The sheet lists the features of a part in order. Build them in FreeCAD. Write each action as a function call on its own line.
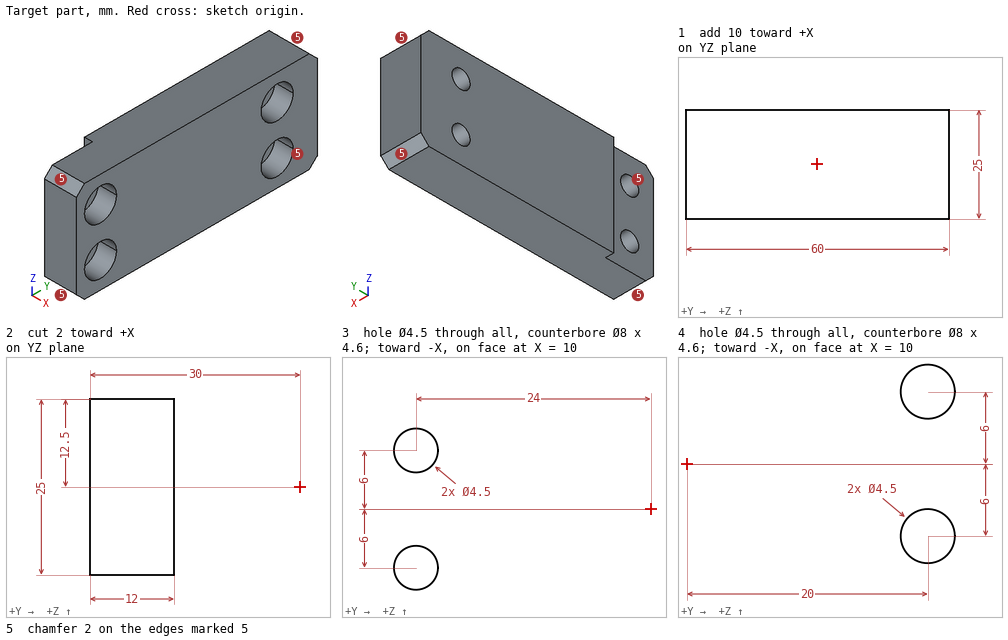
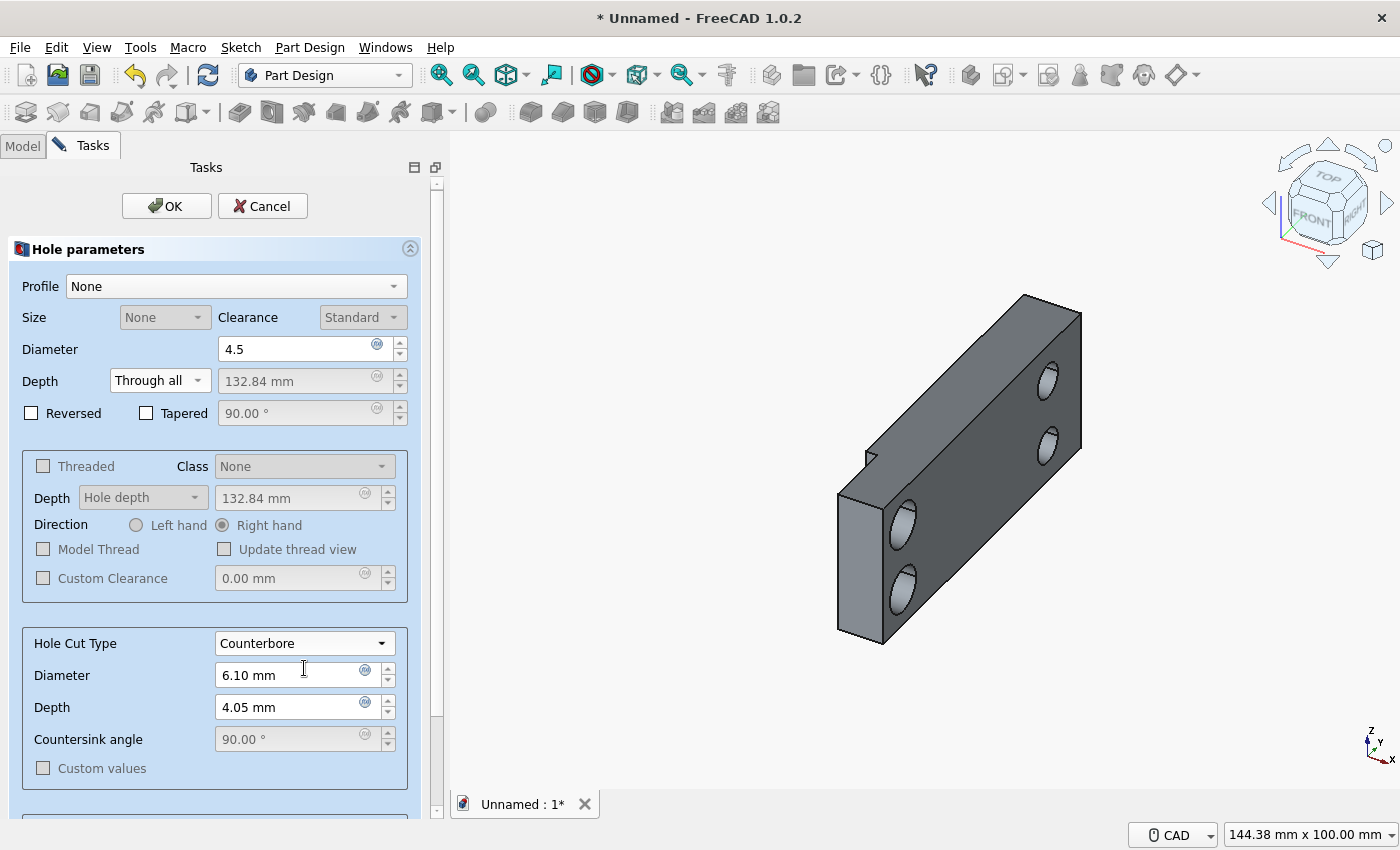
triple_click(298, 675)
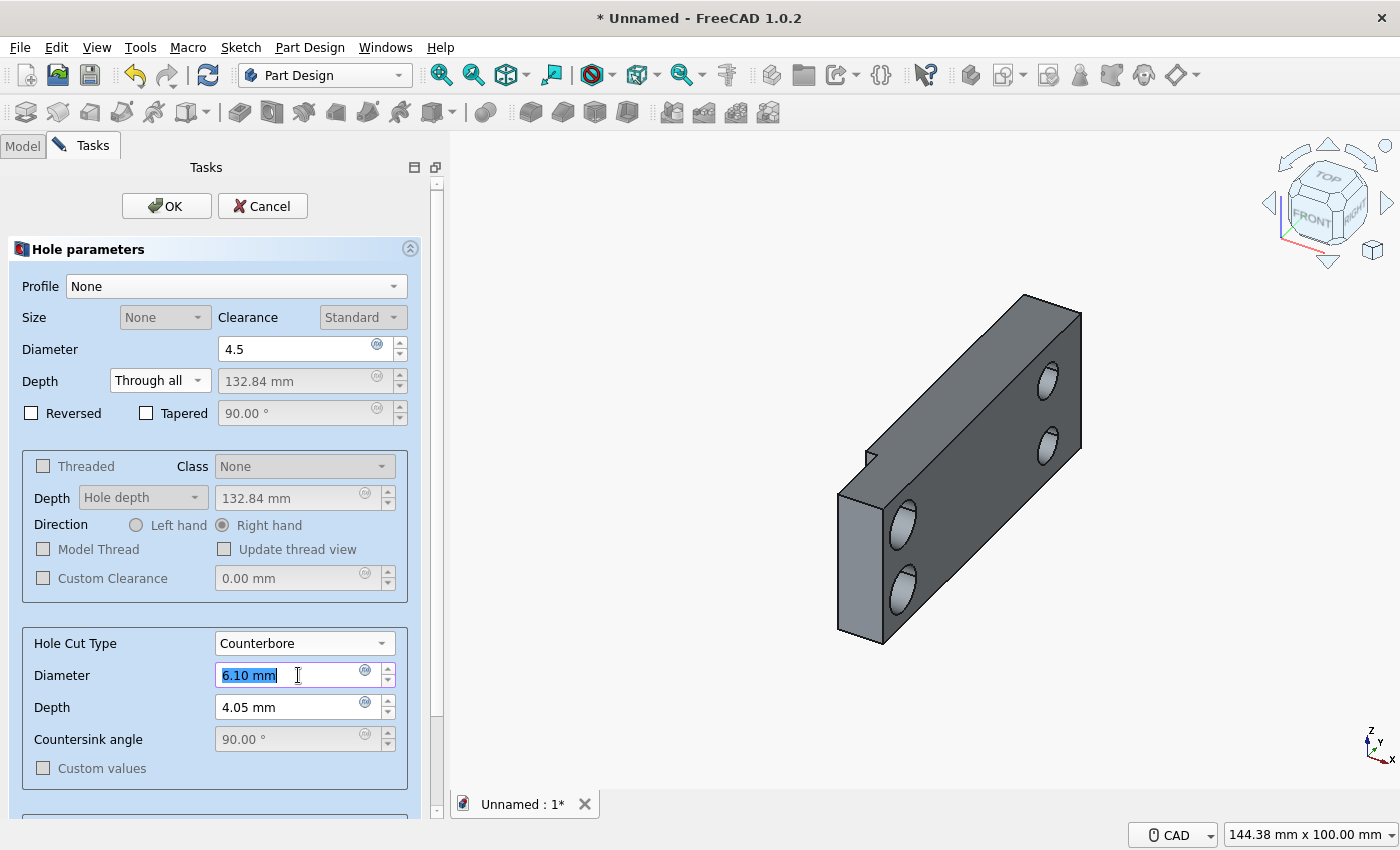
text(8)
key(Tab)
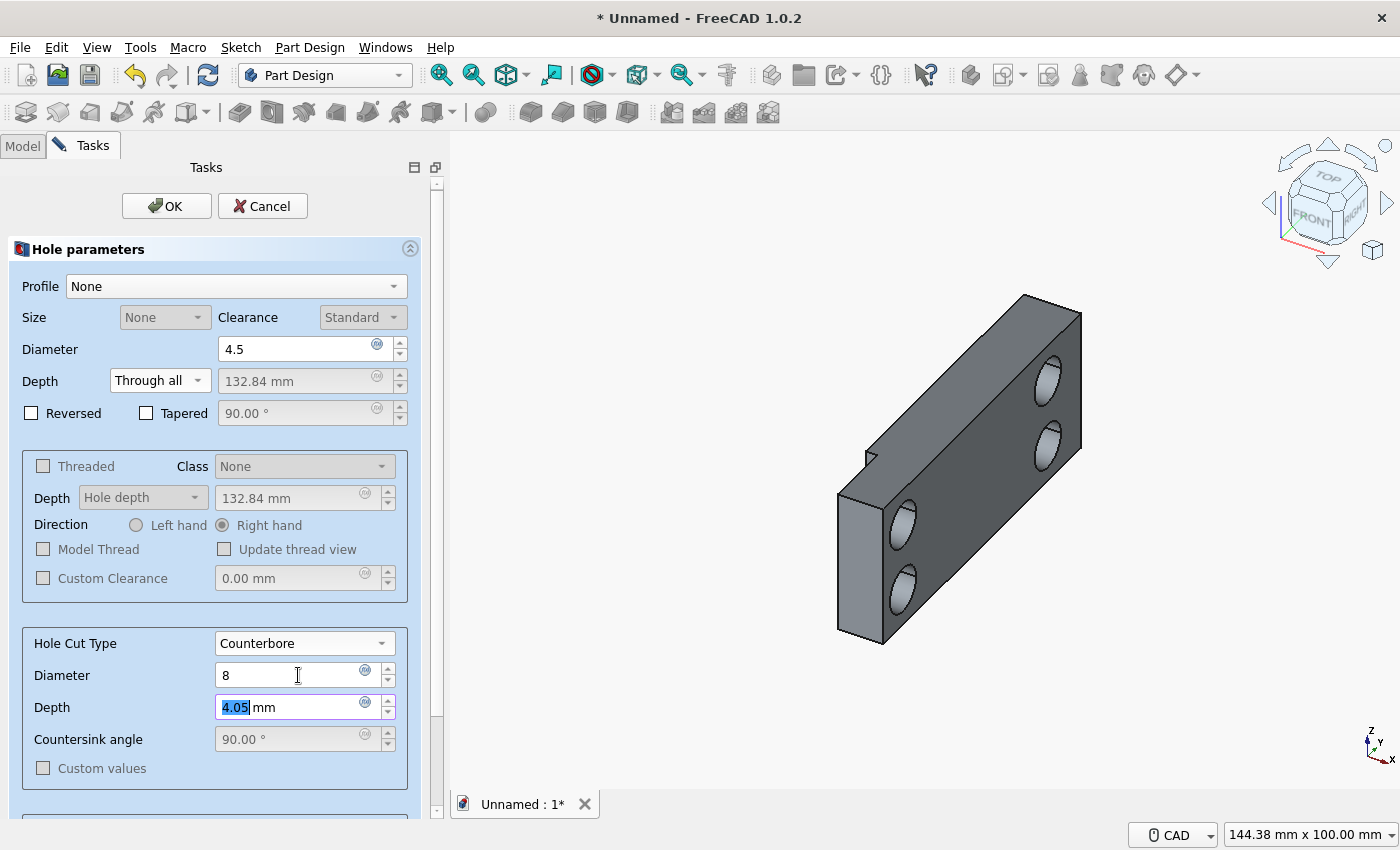
text(4.6)
key(Tab)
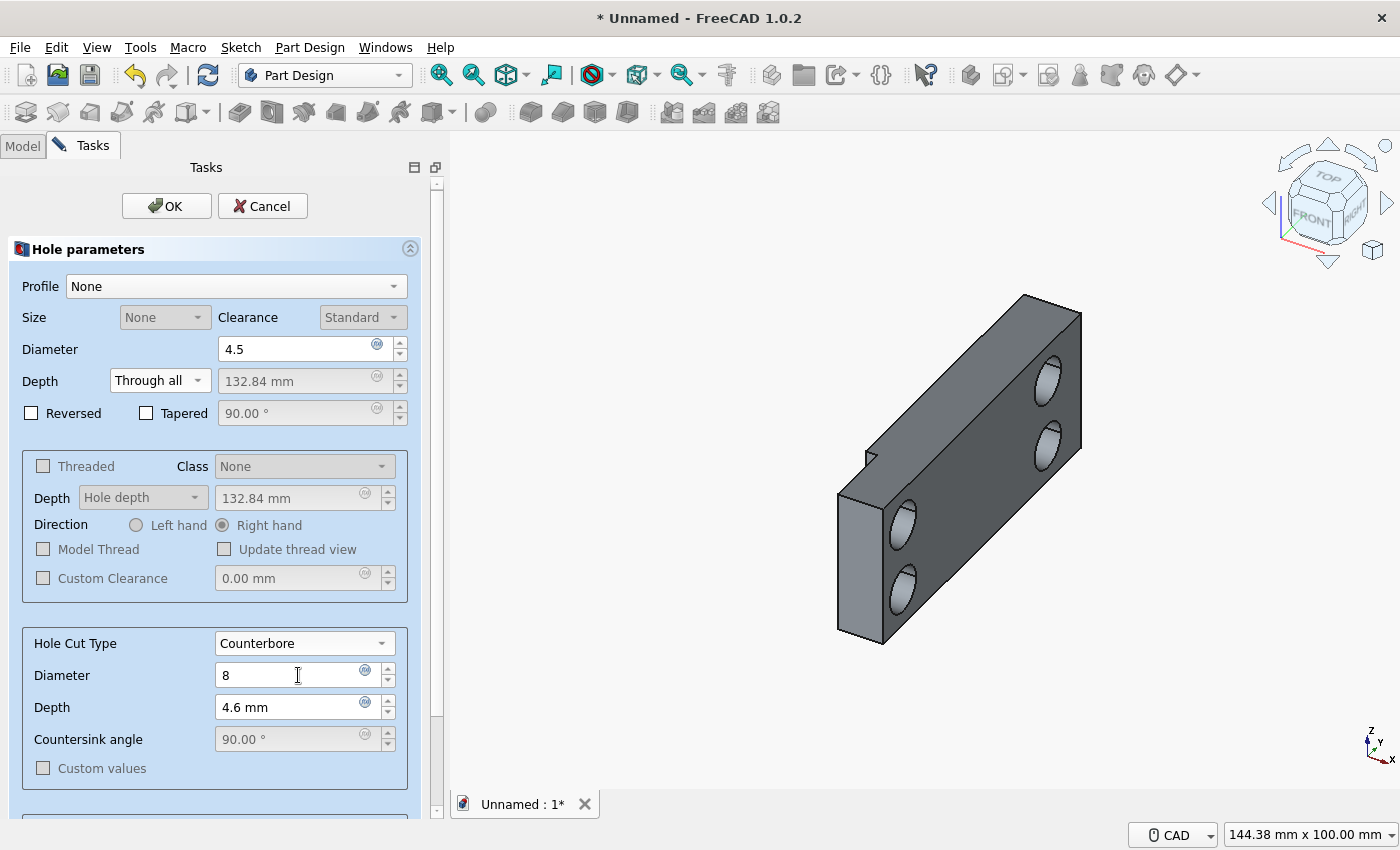
click(167, 206)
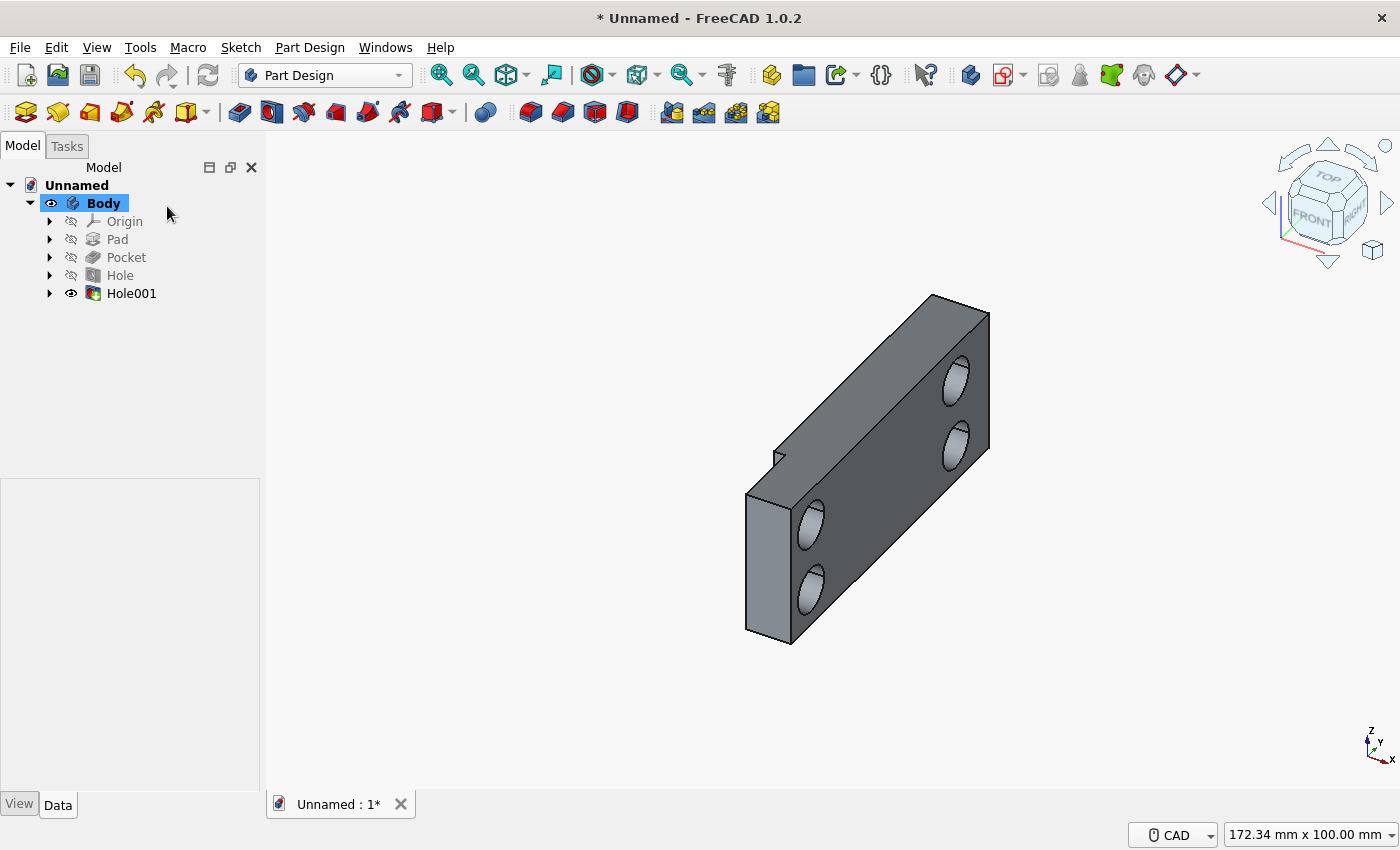
click(768, 501)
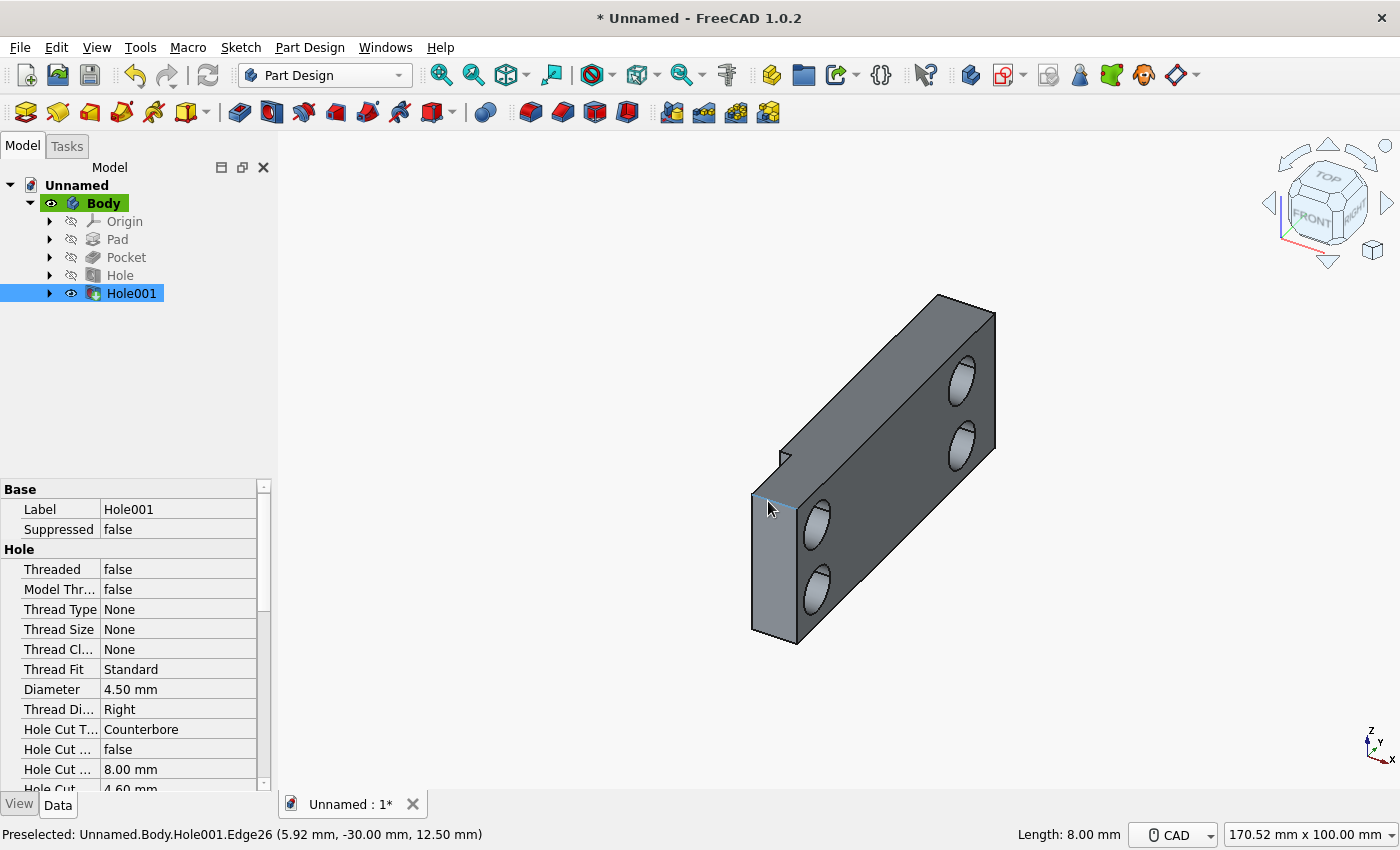
key(0)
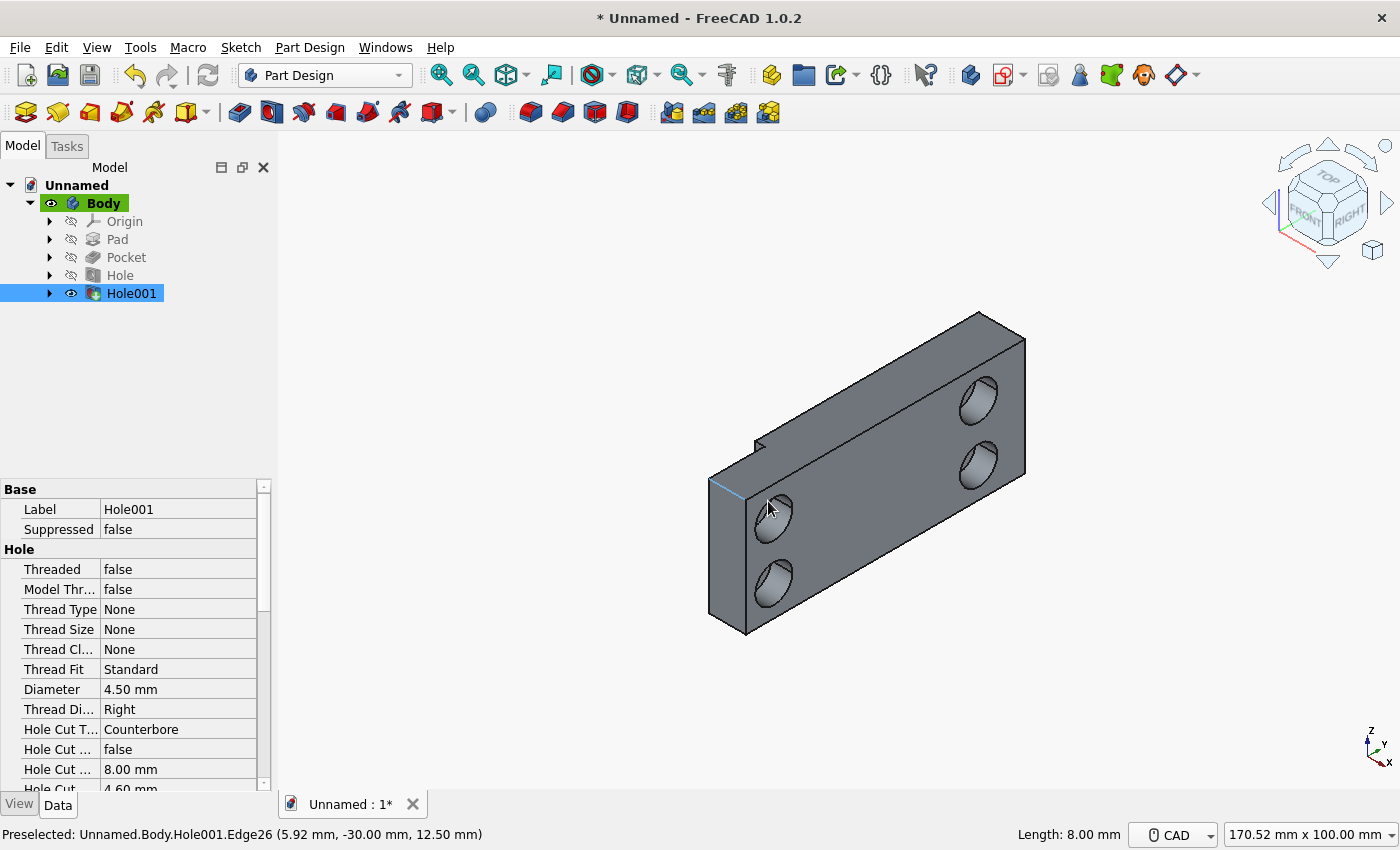
key(2)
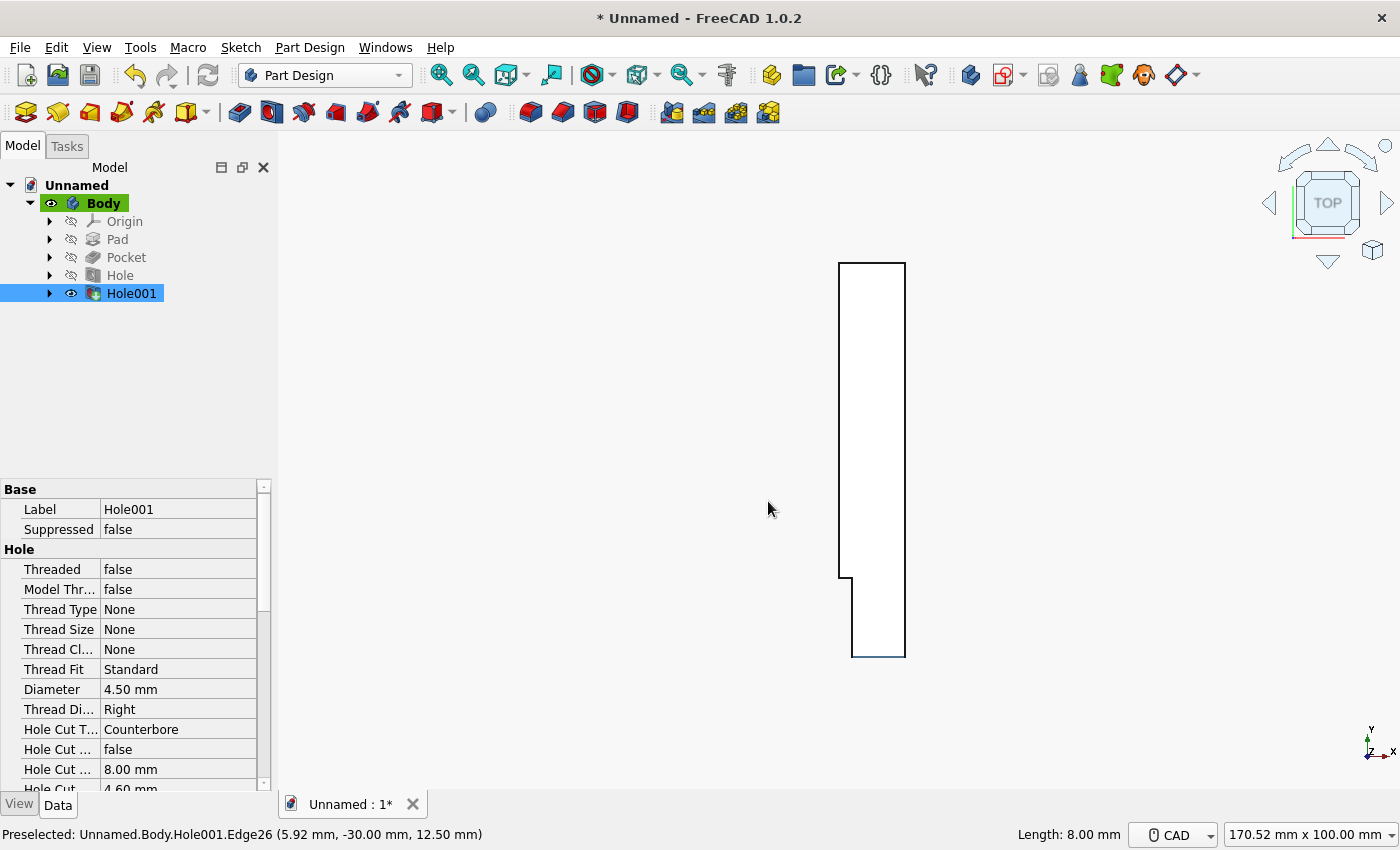
click(872, 262, ctrl)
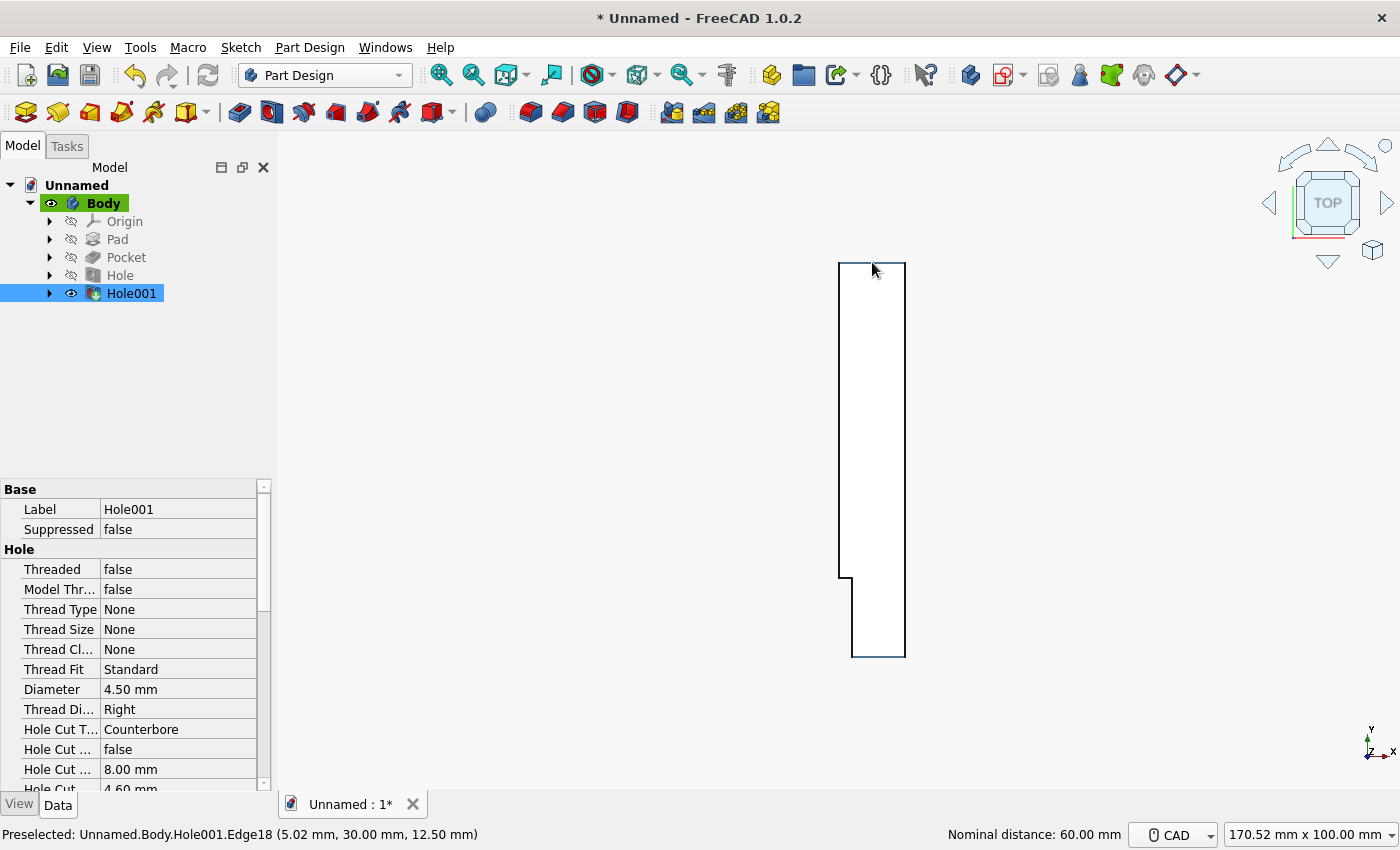
key(1)